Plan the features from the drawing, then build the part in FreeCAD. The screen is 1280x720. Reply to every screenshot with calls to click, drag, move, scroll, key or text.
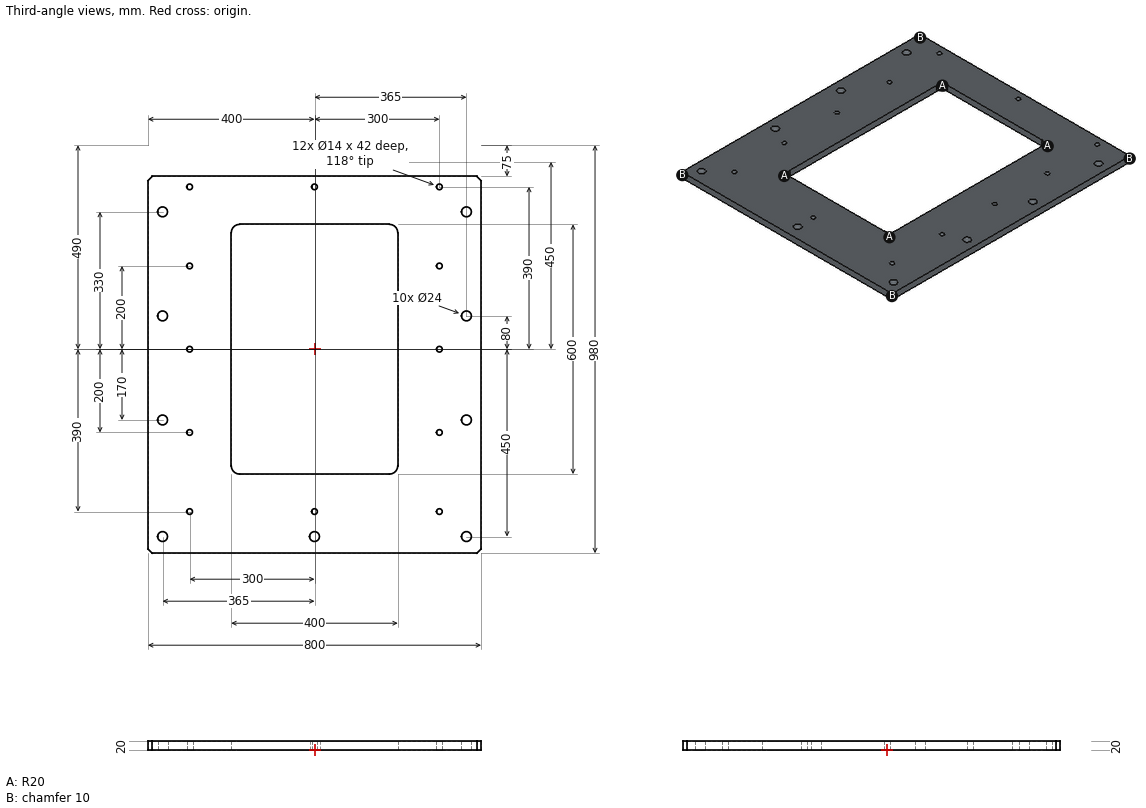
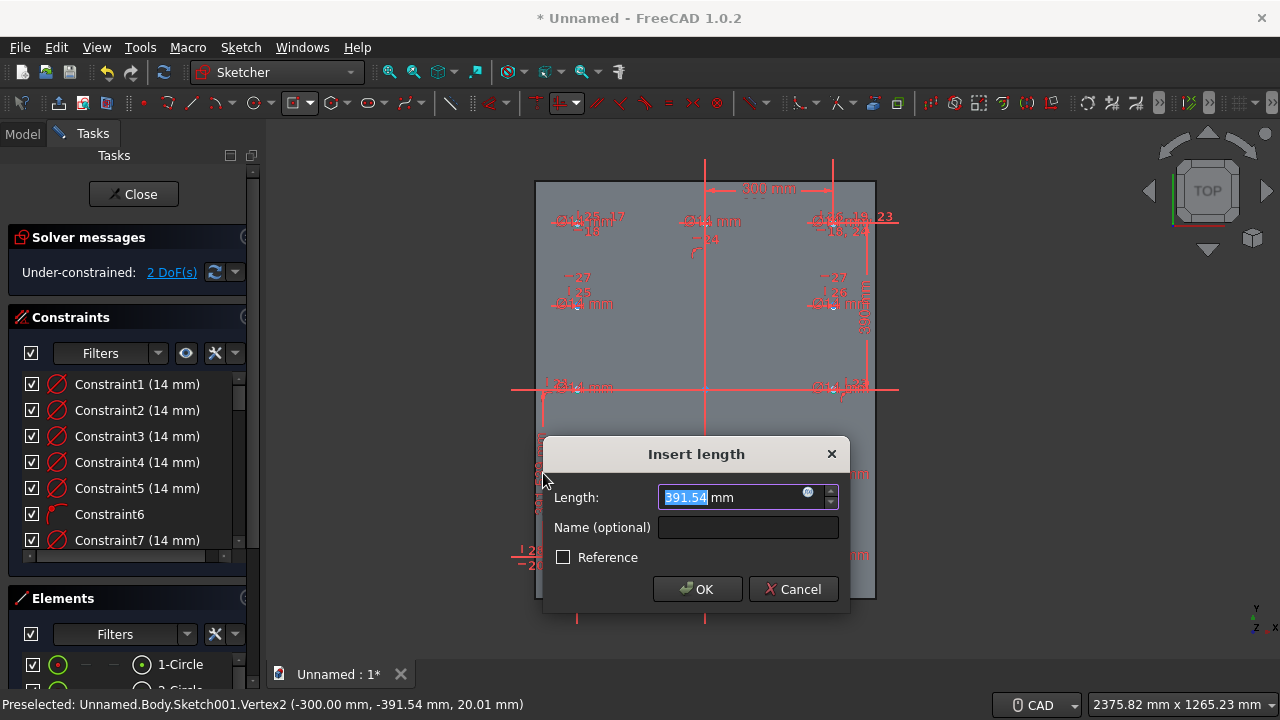
text(390)
key(Return)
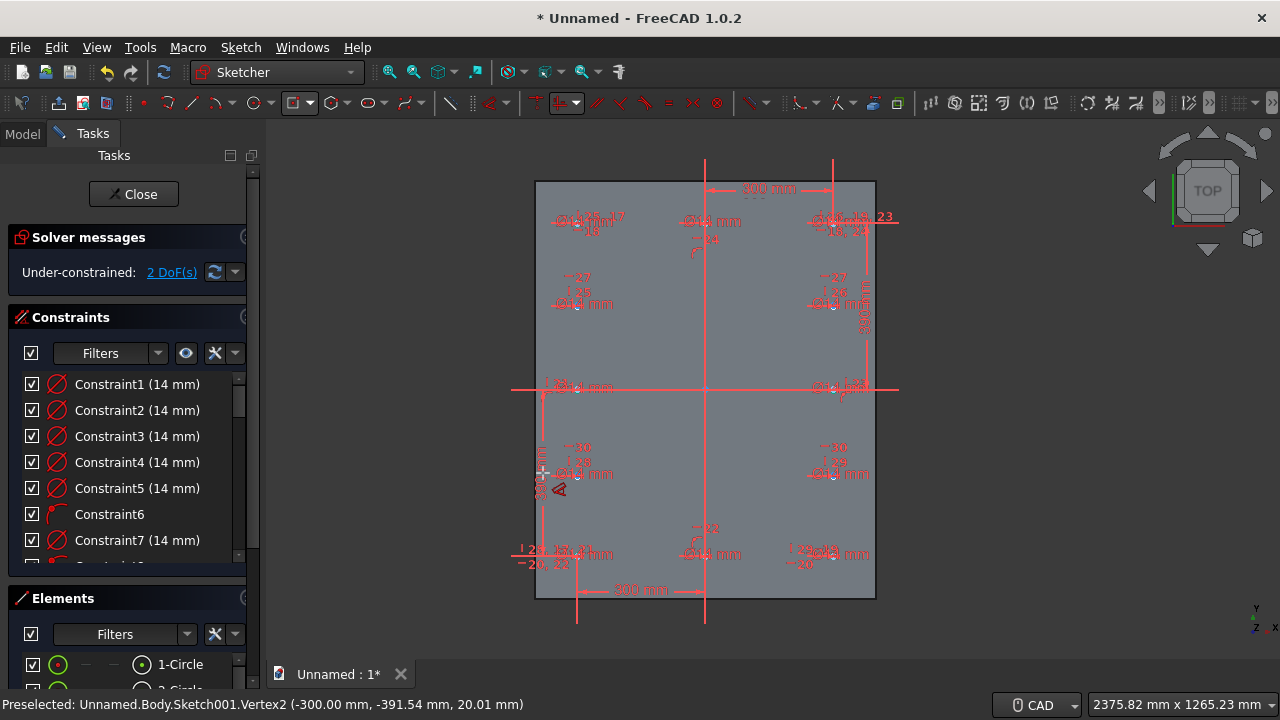
click(577, 306)
click(543, 348)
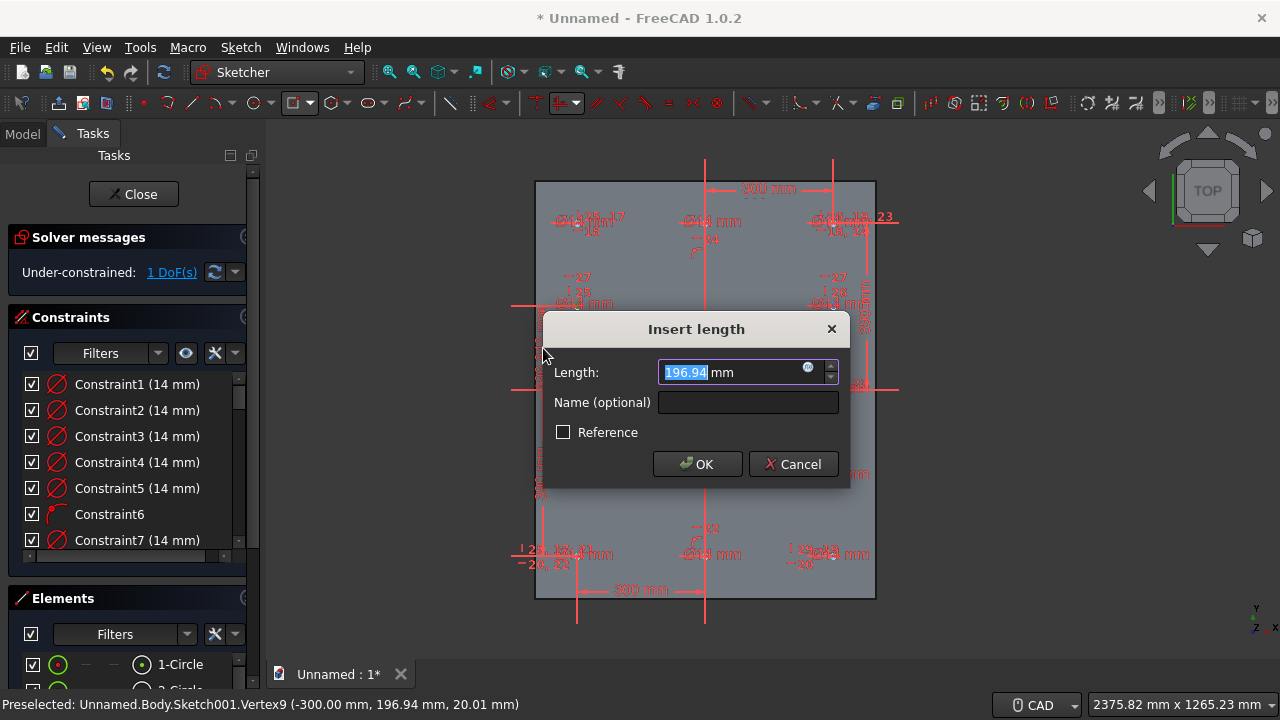
text(200)
key(Return)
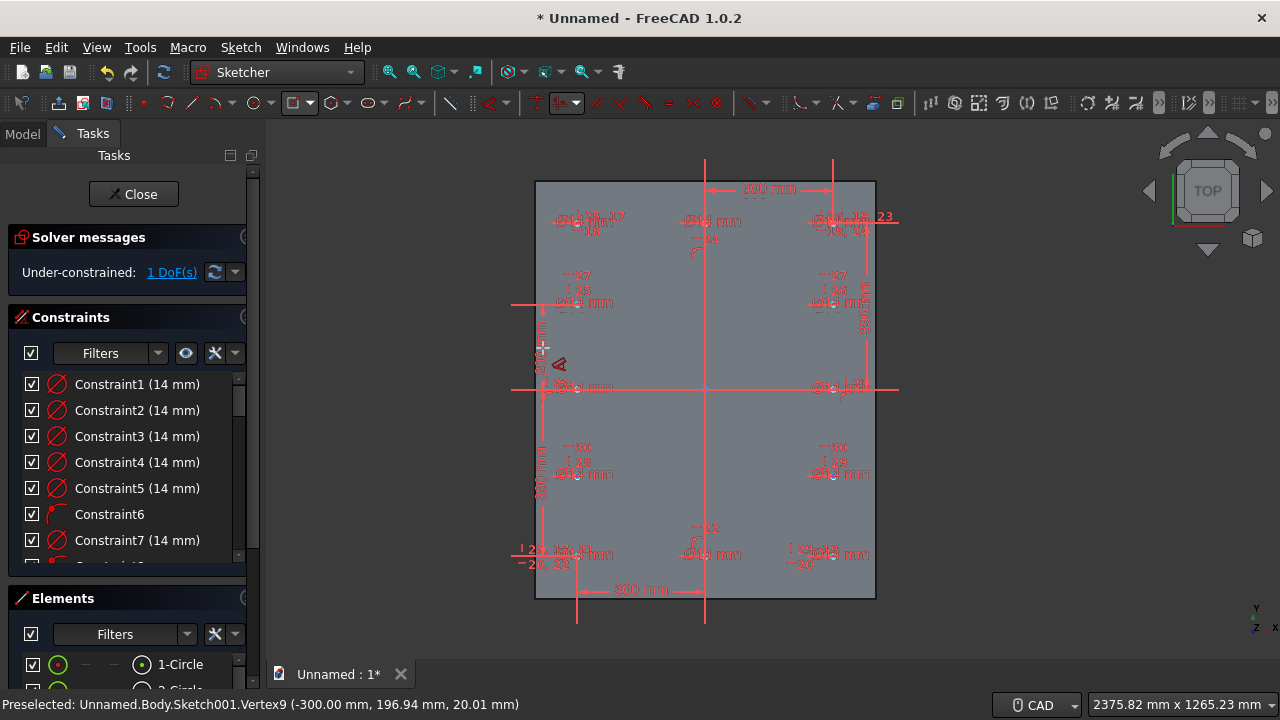
click(577, 476)
click(543, 433)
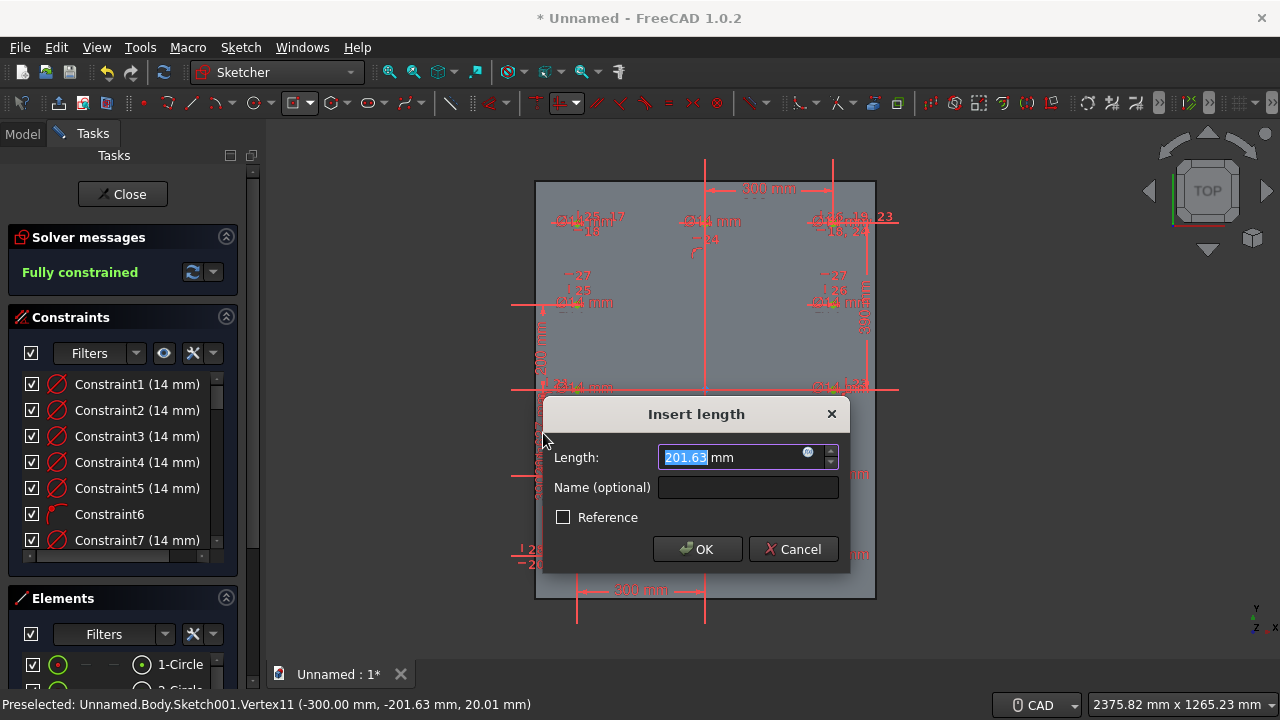
text(200)
key(Return)
key(Escape)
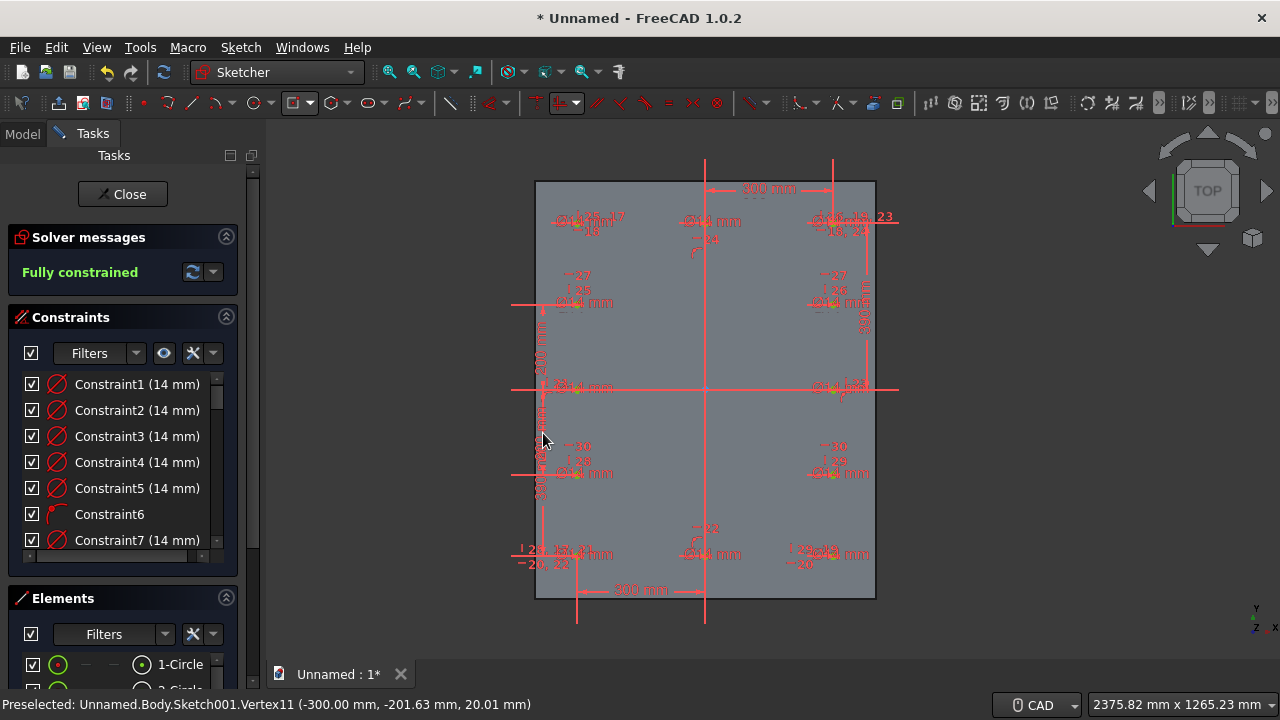
click(123, 194)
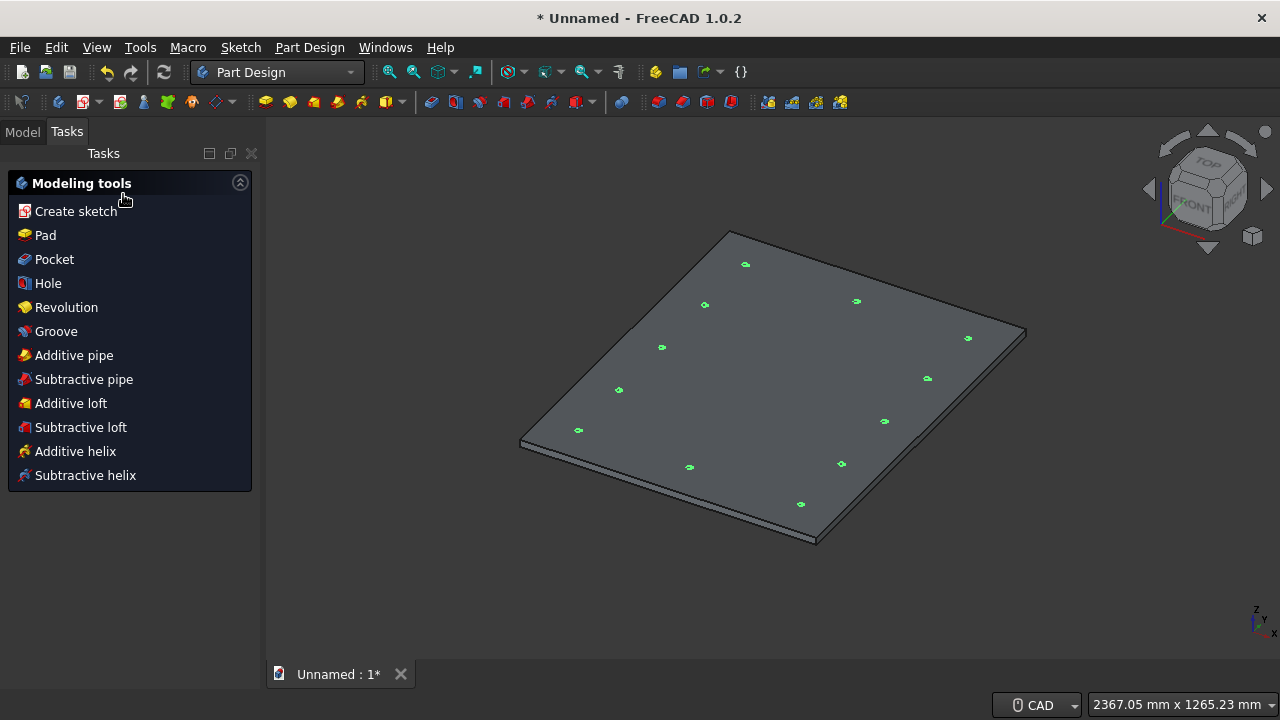
click(456, 102)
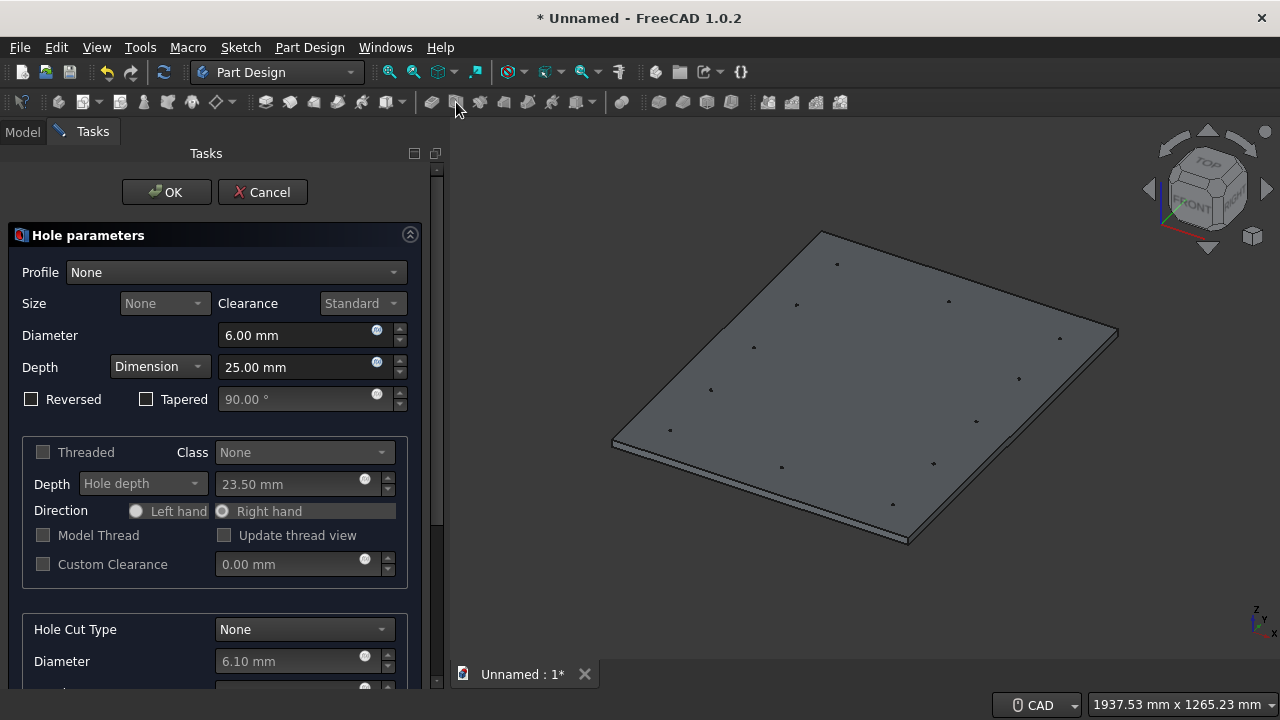
triple_click(305, 335)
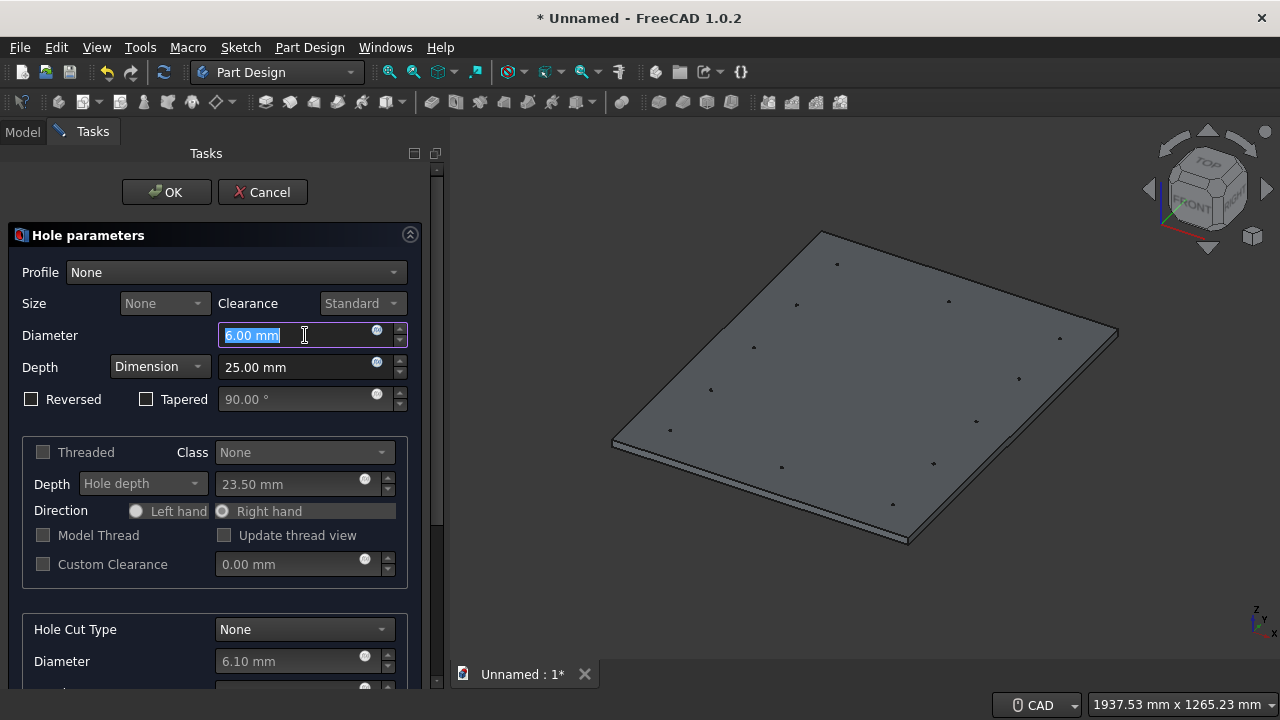
text(14)
key(Tab)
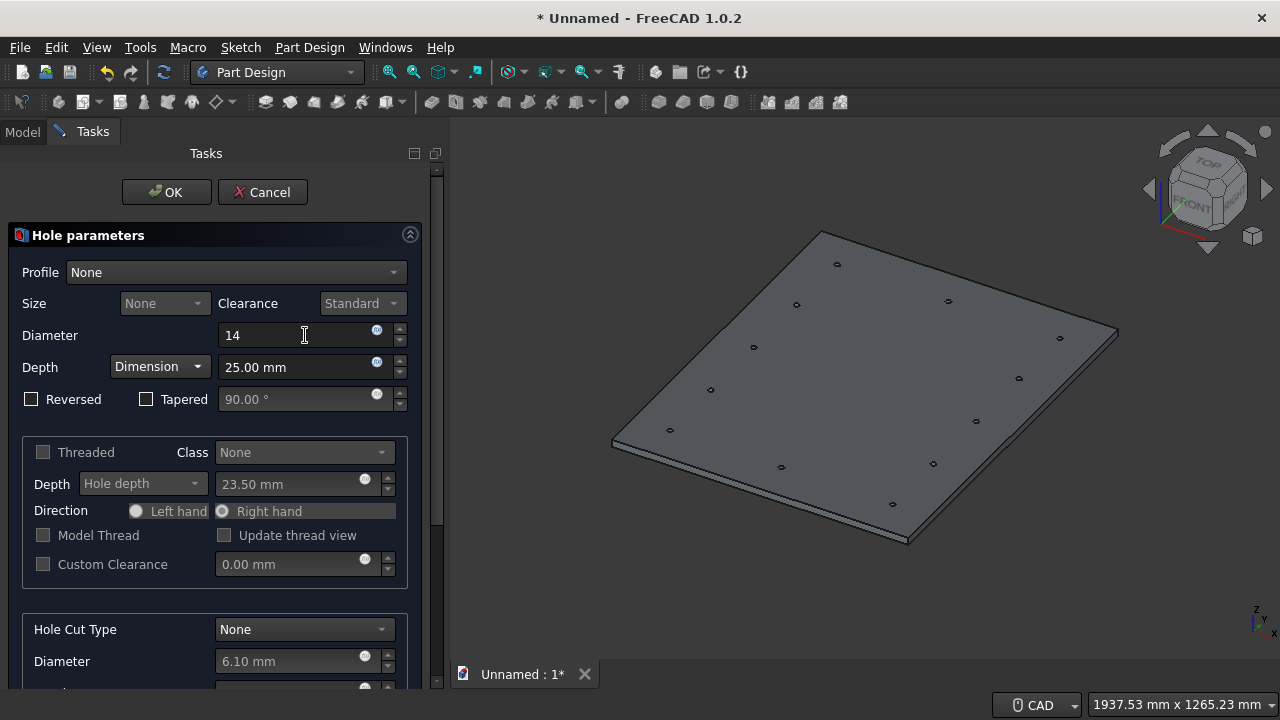
triple_click(305, 367)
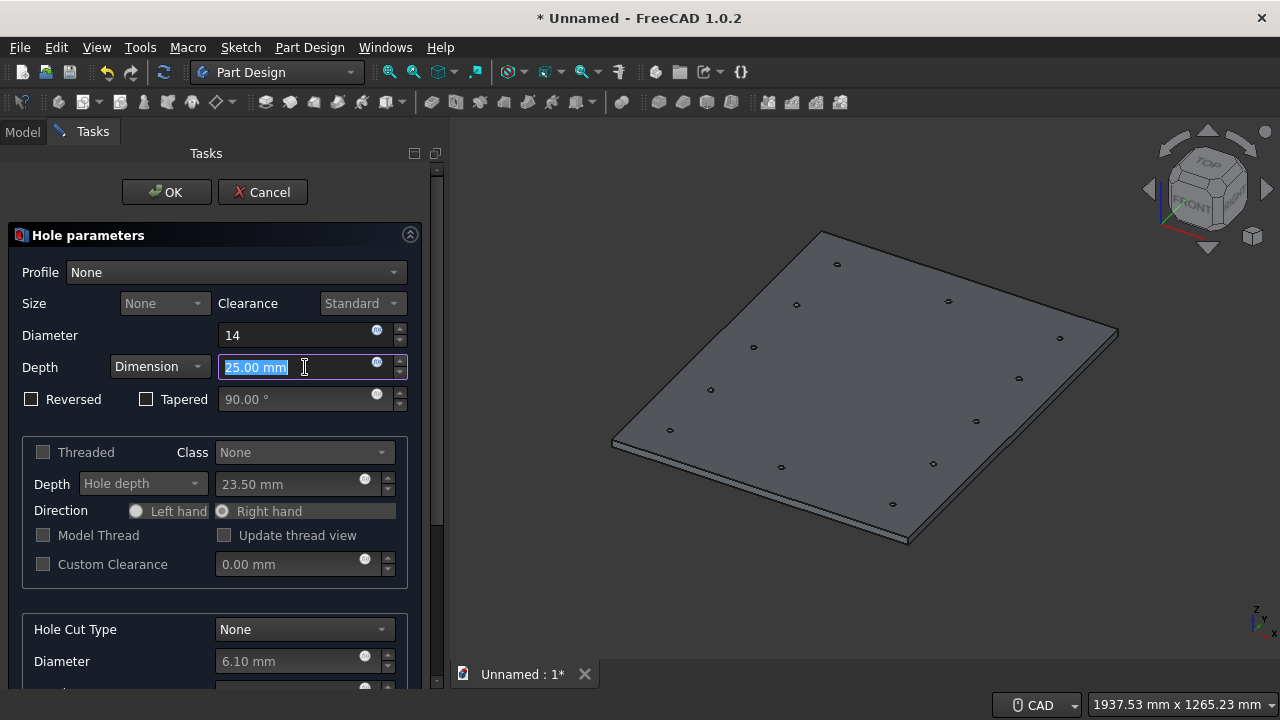
text(42)
key(Tab)